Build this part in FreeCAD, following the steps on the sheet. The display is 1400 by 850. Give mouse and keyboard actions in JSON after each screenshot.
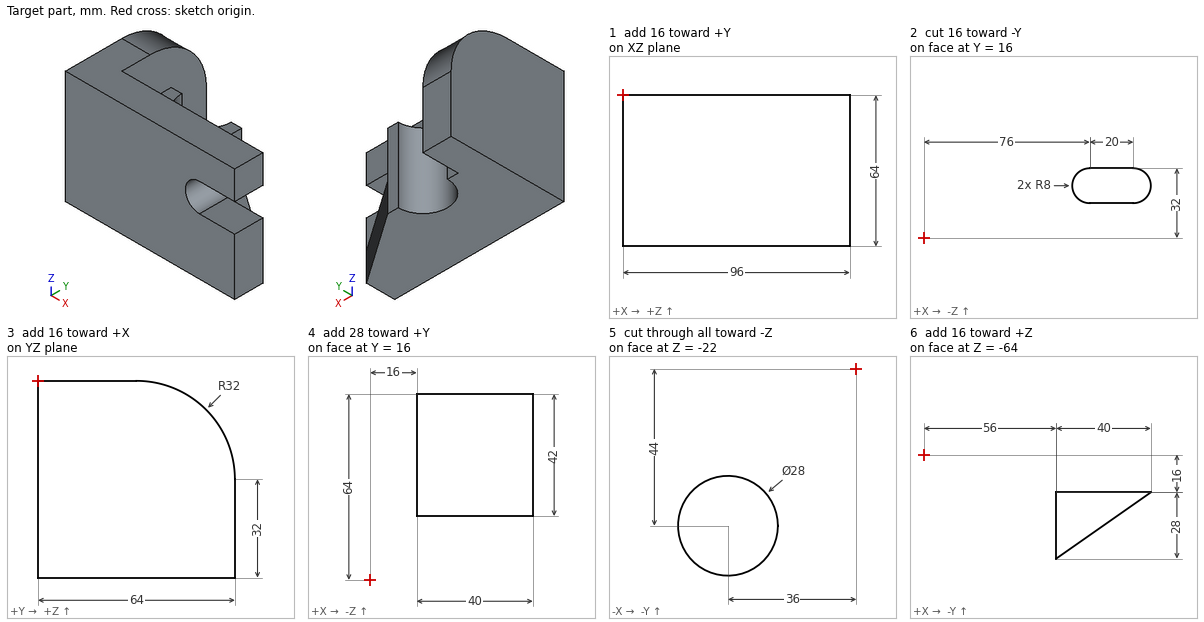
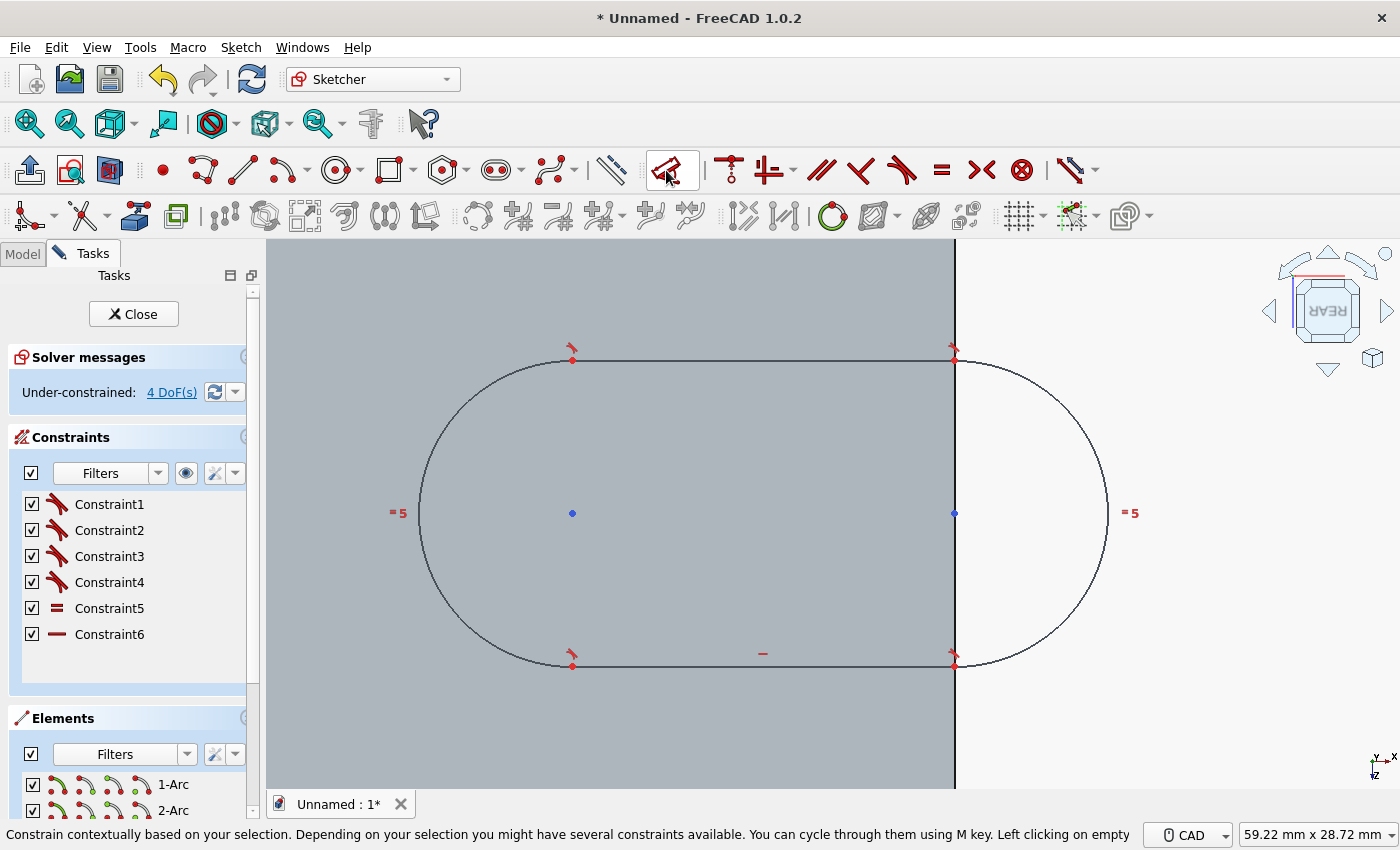
{"action": "left_click", "coordinate": [448, 424]}
{"action": "left_click", "coordinate": [422, 405]}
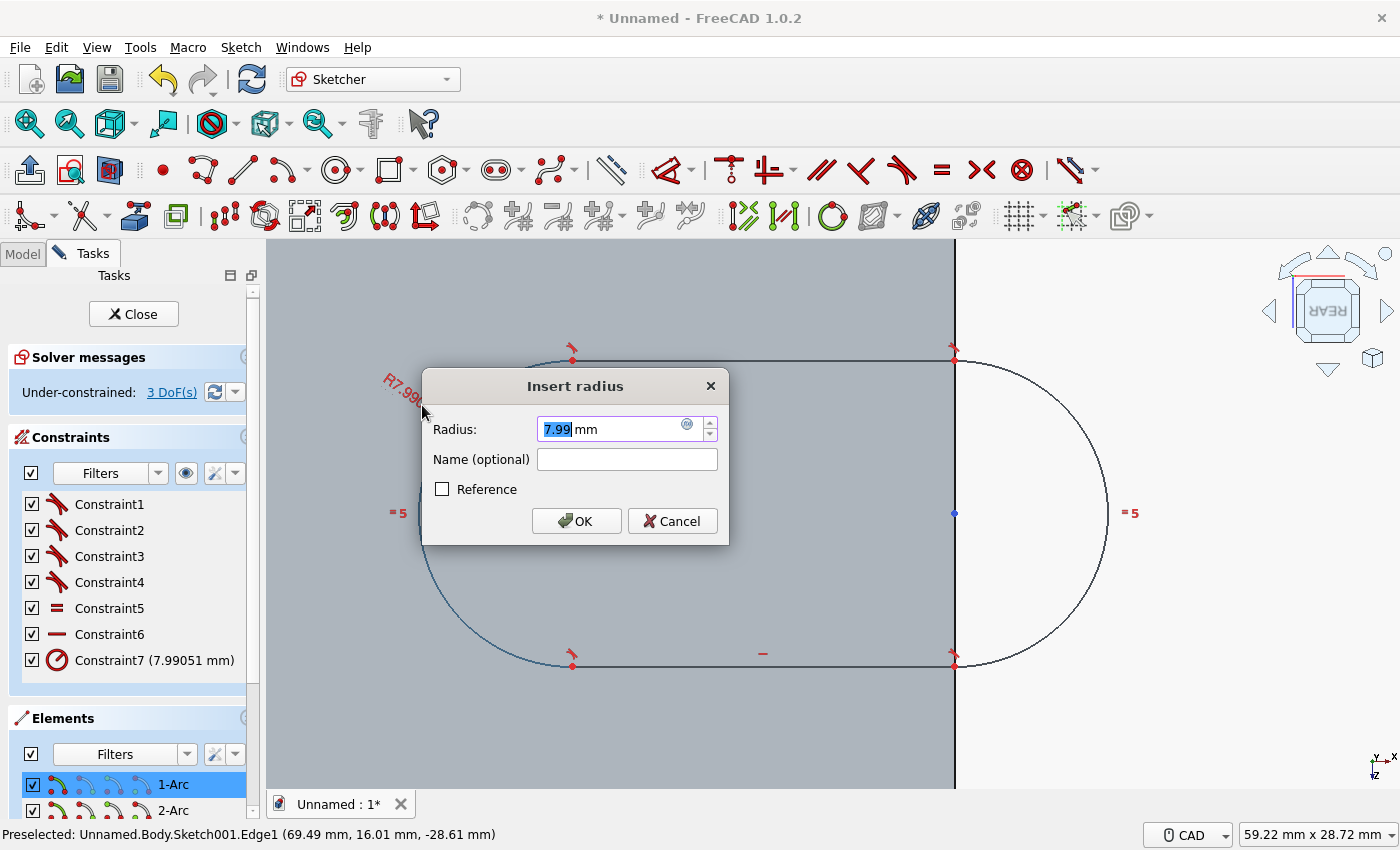
{"action": "type", "text": "8"}
{"action": "key", "text": "Return"}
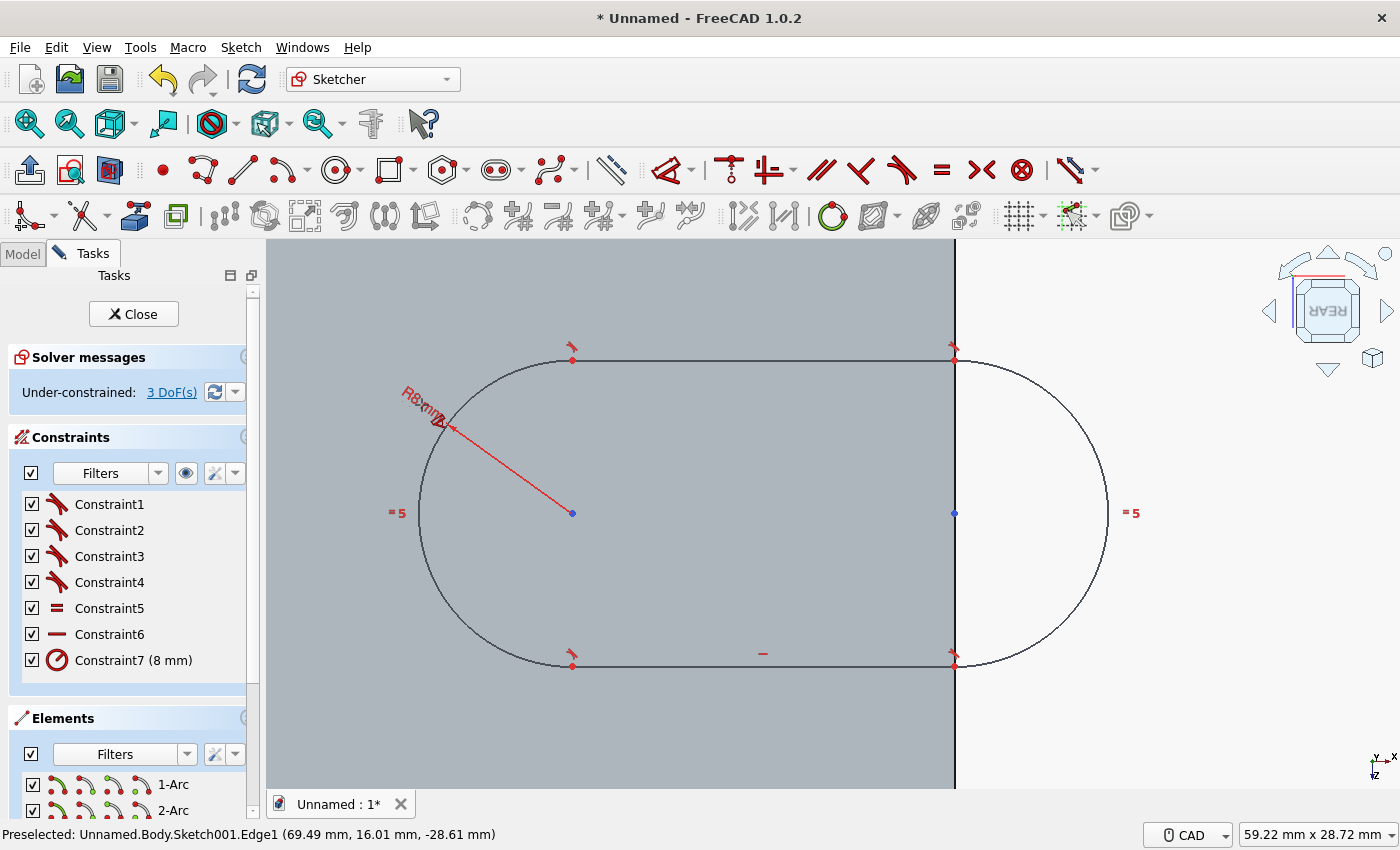
{"action": "left_click", "coordinate": [687, 361]}
{"action": "left_click", "coordinate": [763, 327]}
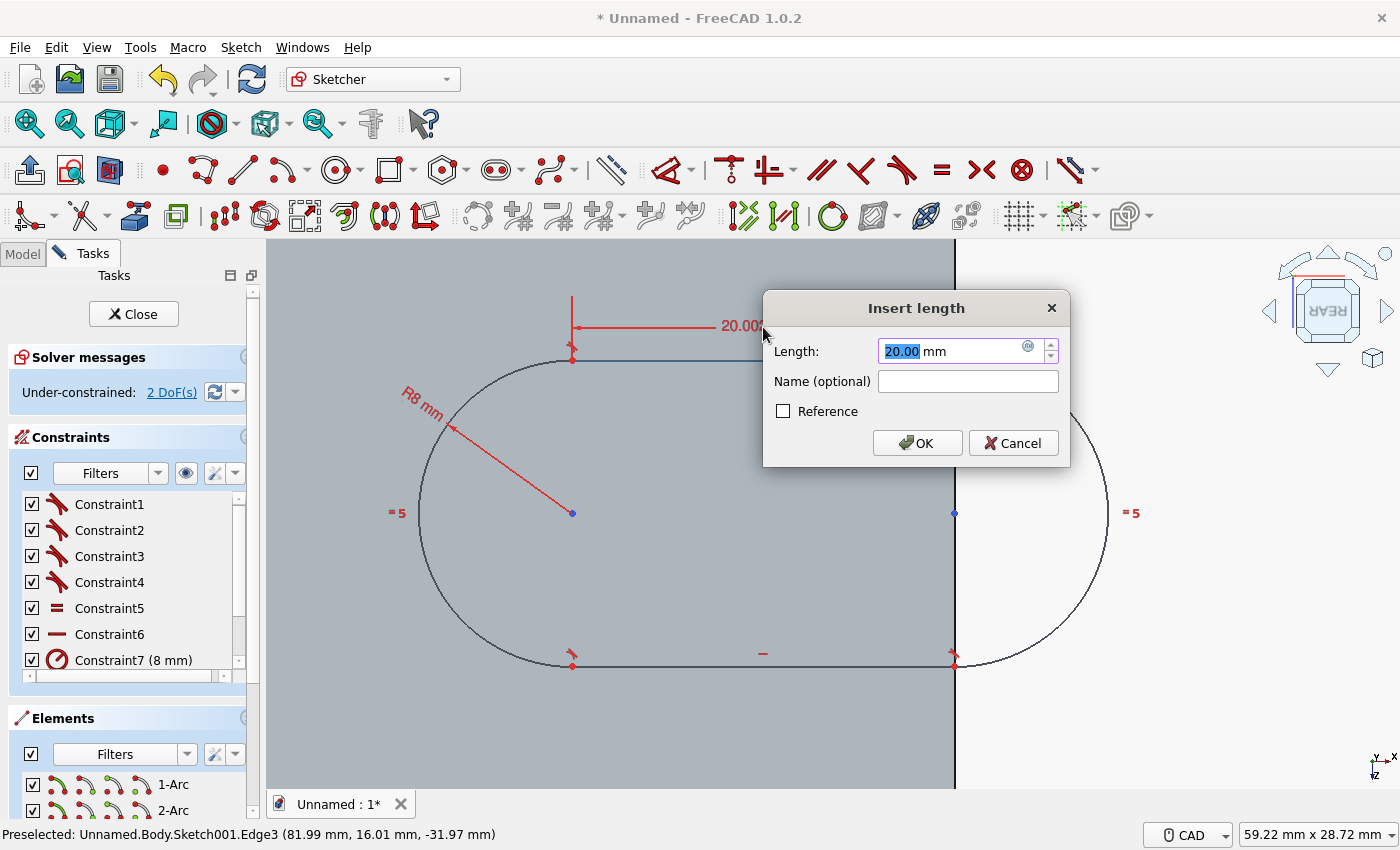
{"action": "type", "text": "20"}
{"action": "key", "text": "Return"}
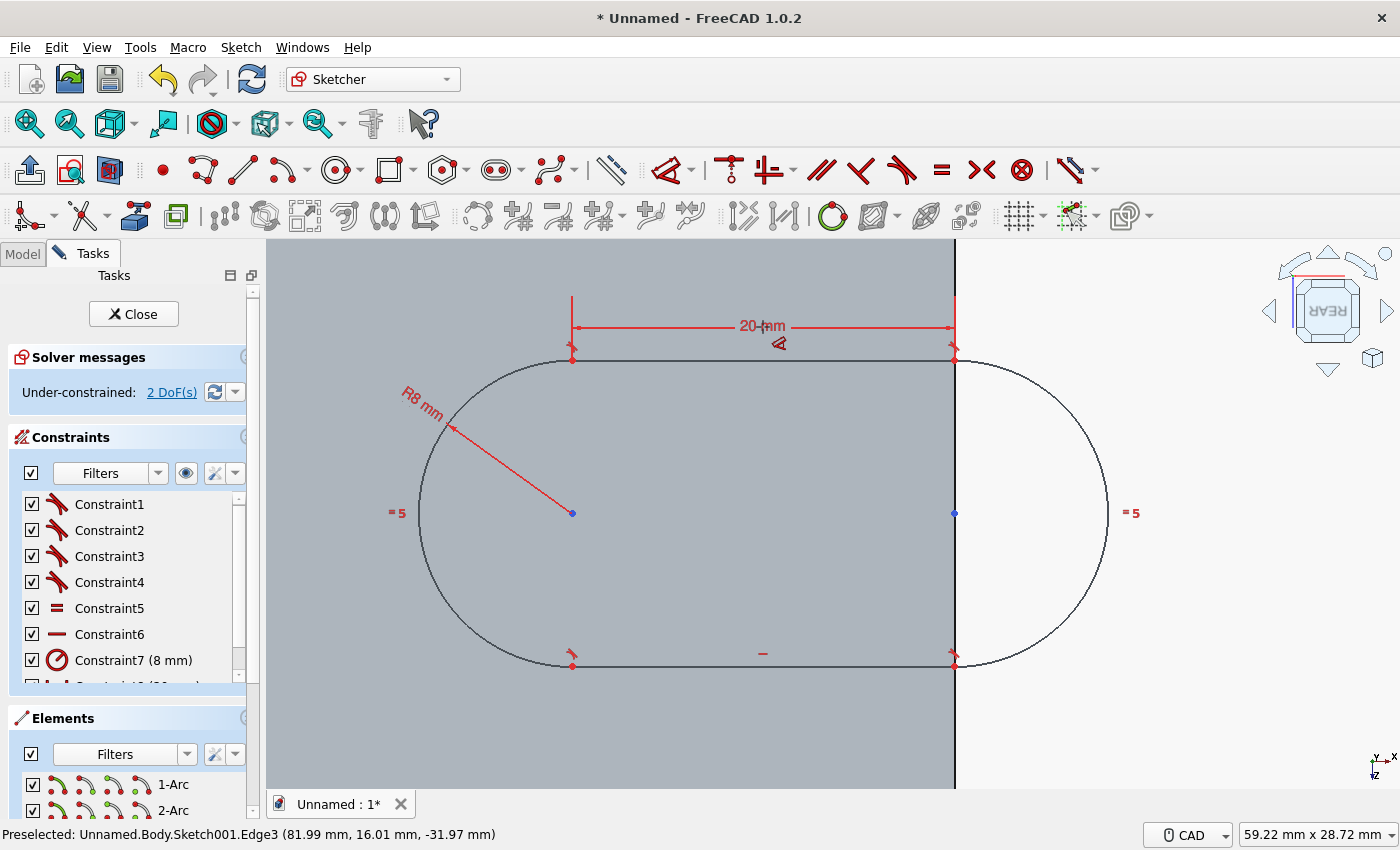
{"action": "left_click", "coordinate": [572, 361]}
{"action": "left_click", "coordinate": [433, 327]}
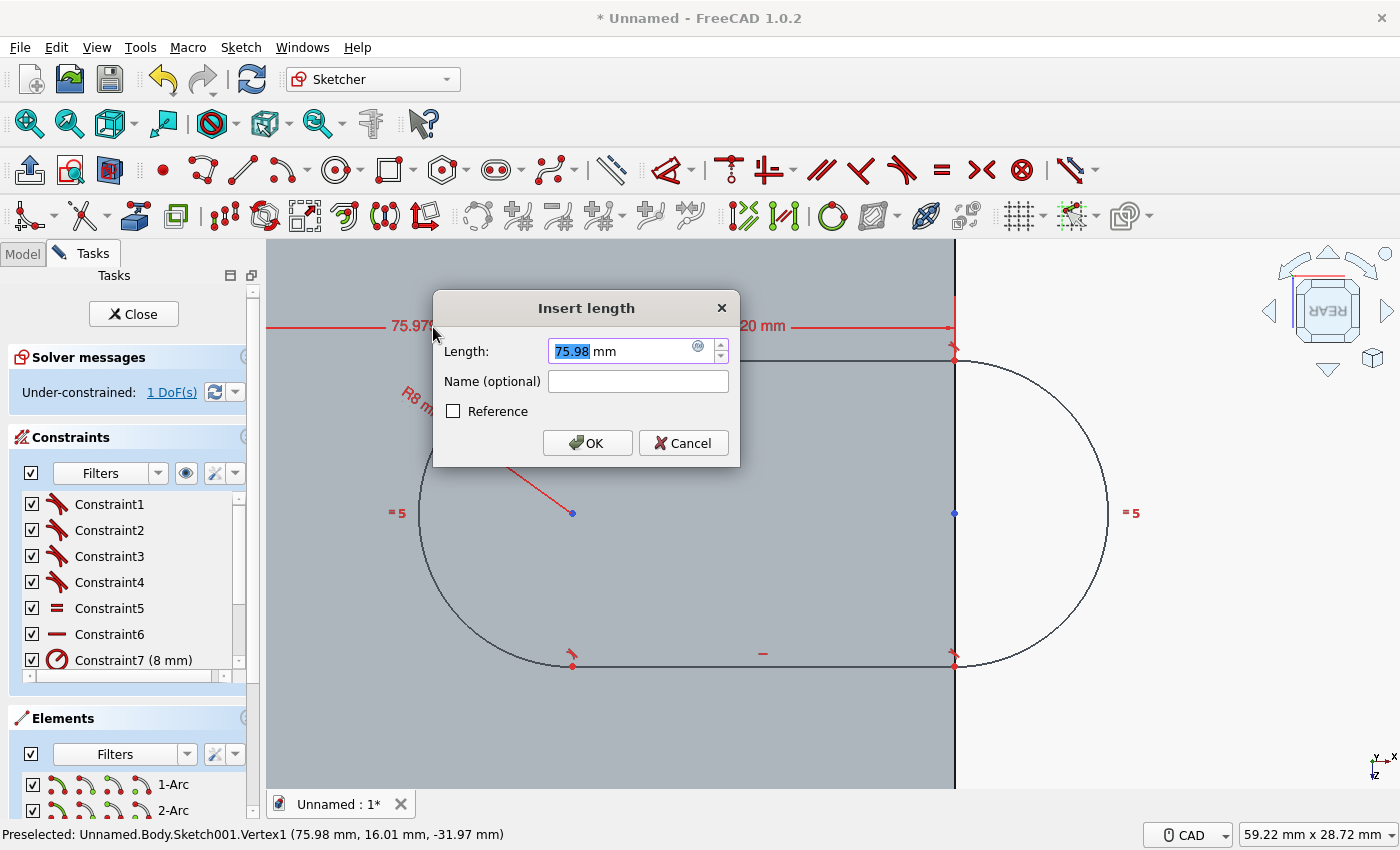
{"action": "type", "text": "76"}
{"action": "key", "text": "Return"}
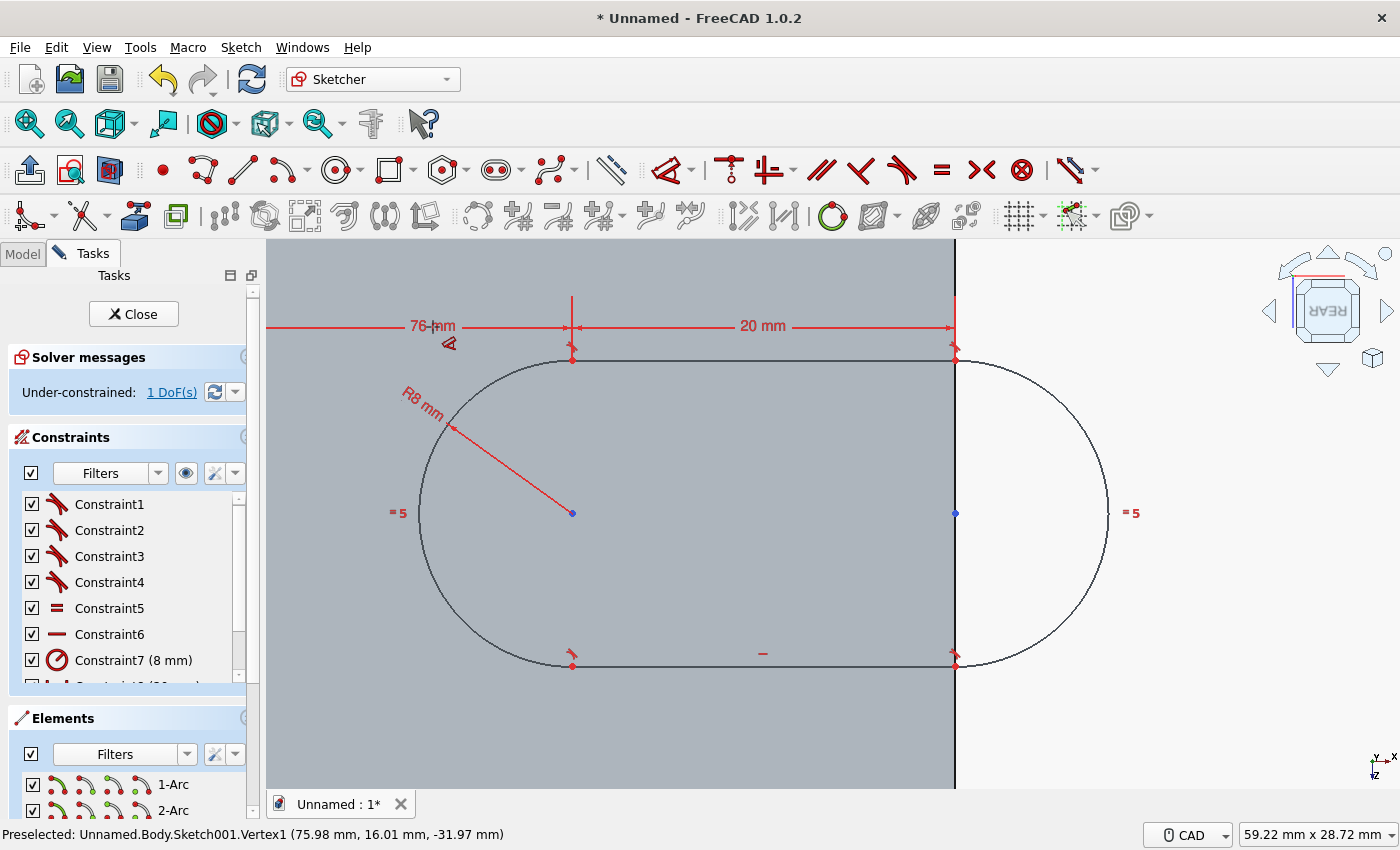
{"action": "left_click", "coordinate": [572, 361]}
{"action": "left_click", "coordinate": [606, 561]}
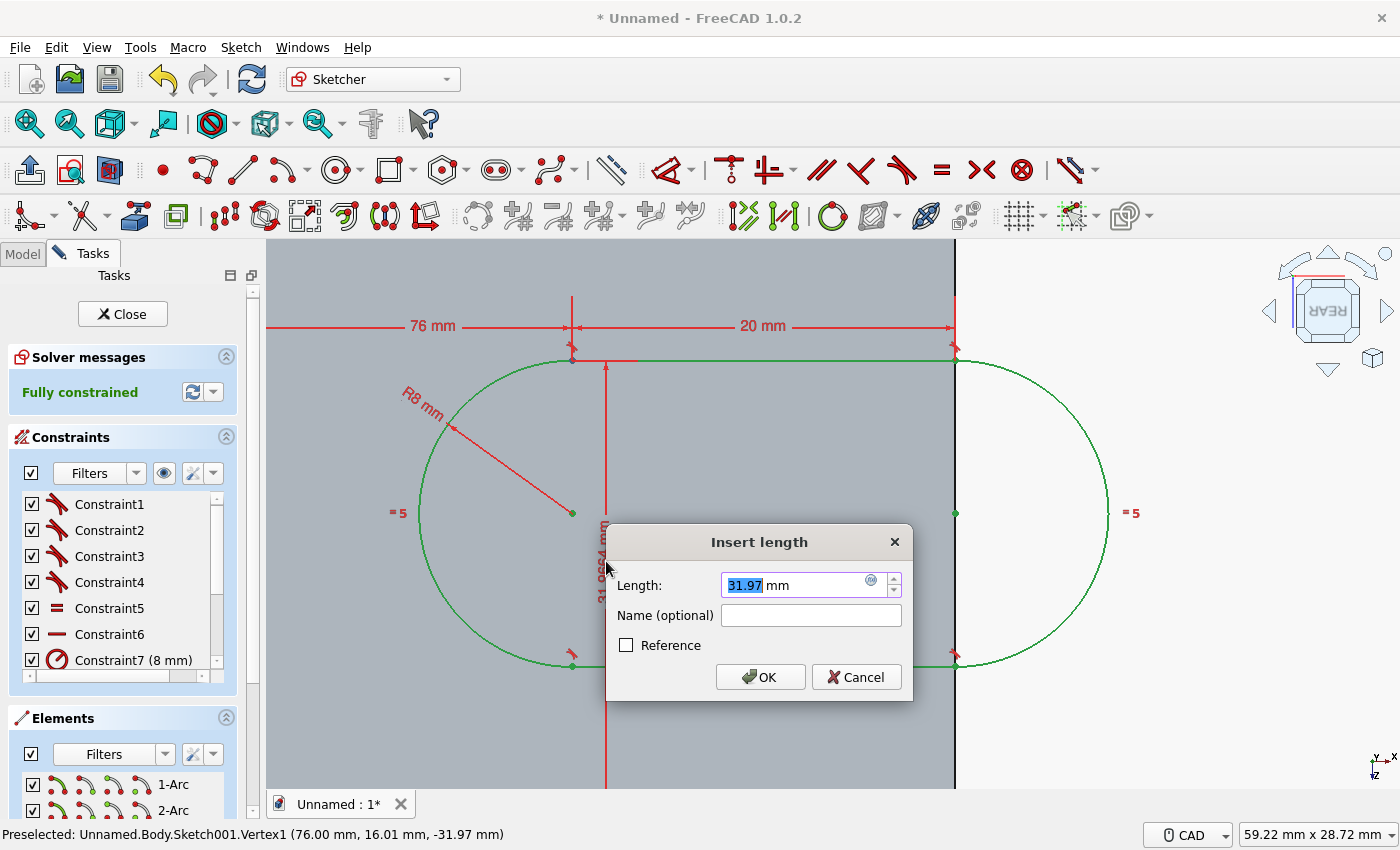
{"action": "type", "text": "32"}
{"action": "key", "text": "Return"}
{"action": "key", "text": "Escape"}